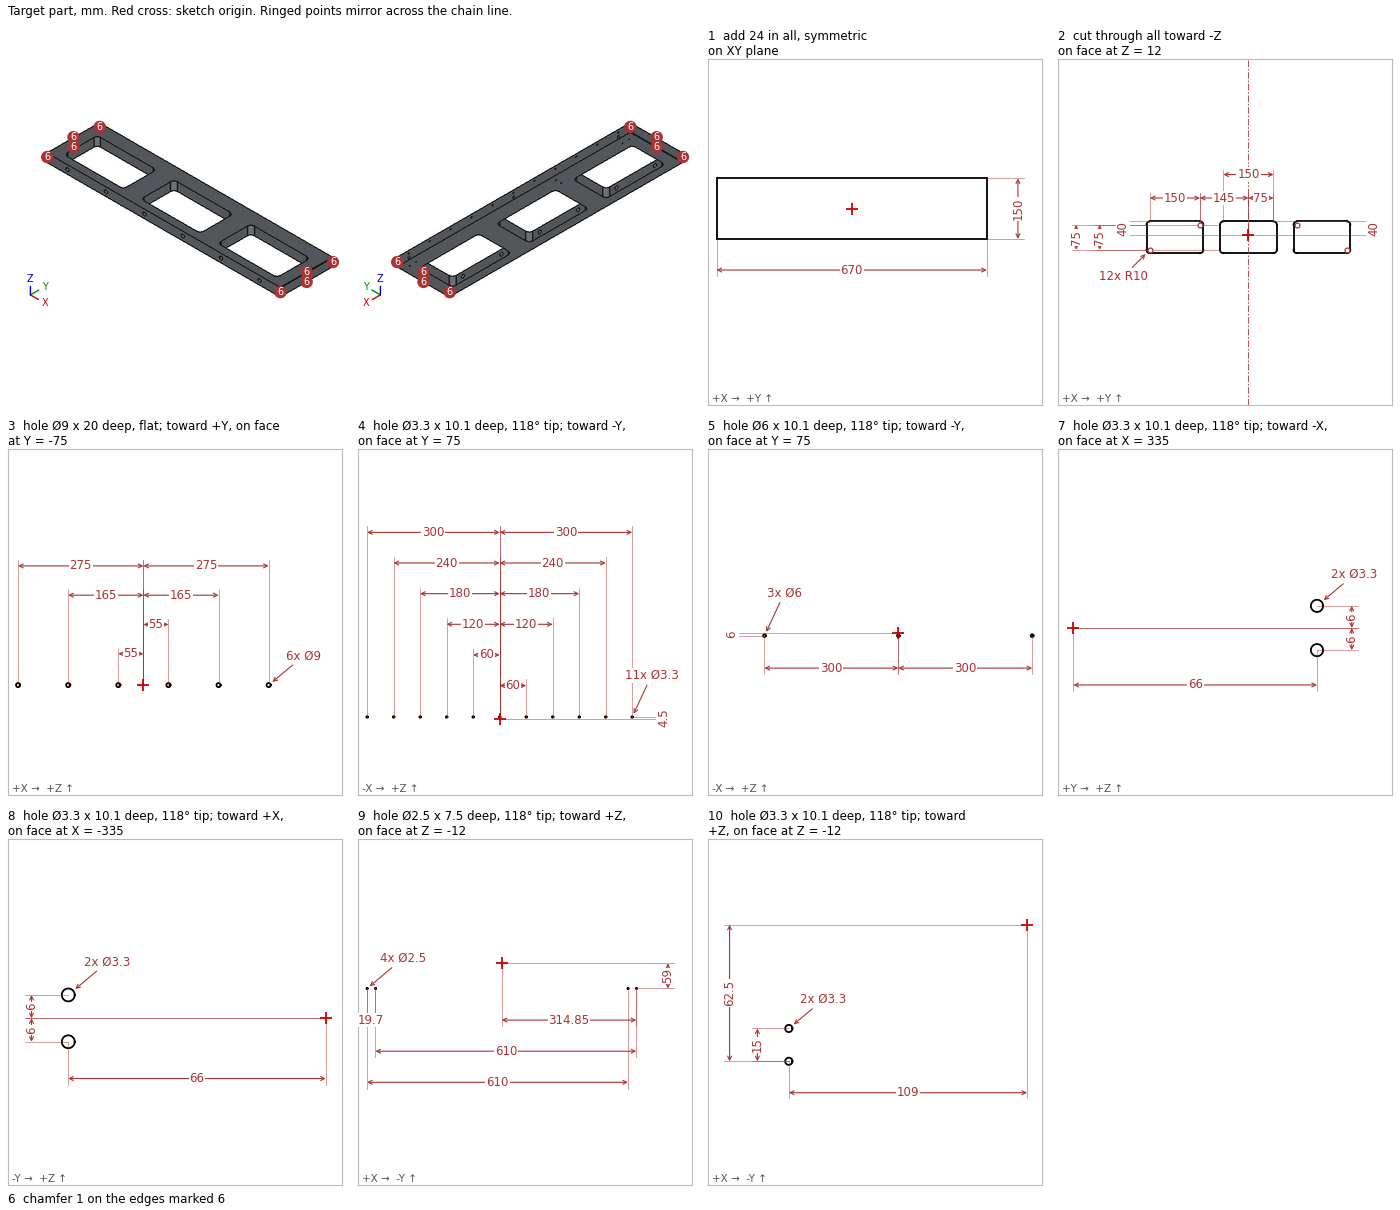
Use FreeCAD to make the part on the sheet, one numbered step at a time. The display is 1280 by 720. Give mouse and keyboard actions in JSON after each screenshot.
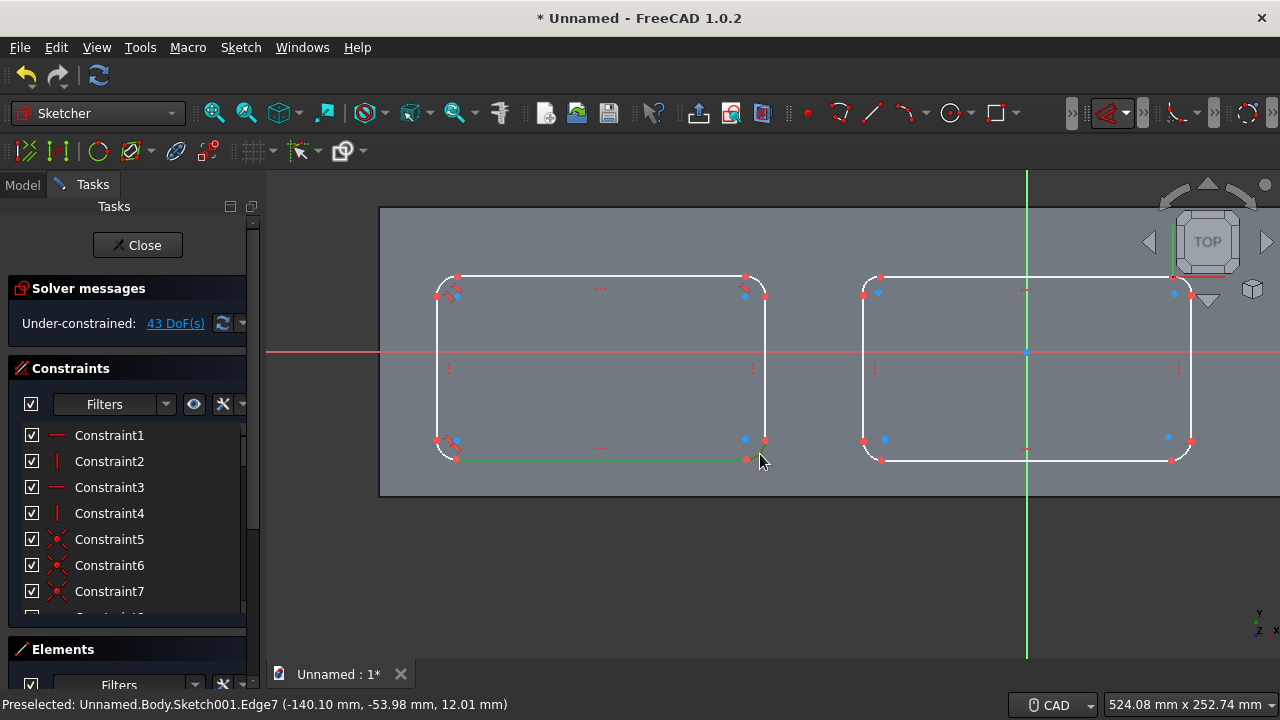
{"action": "key", "text": "t"}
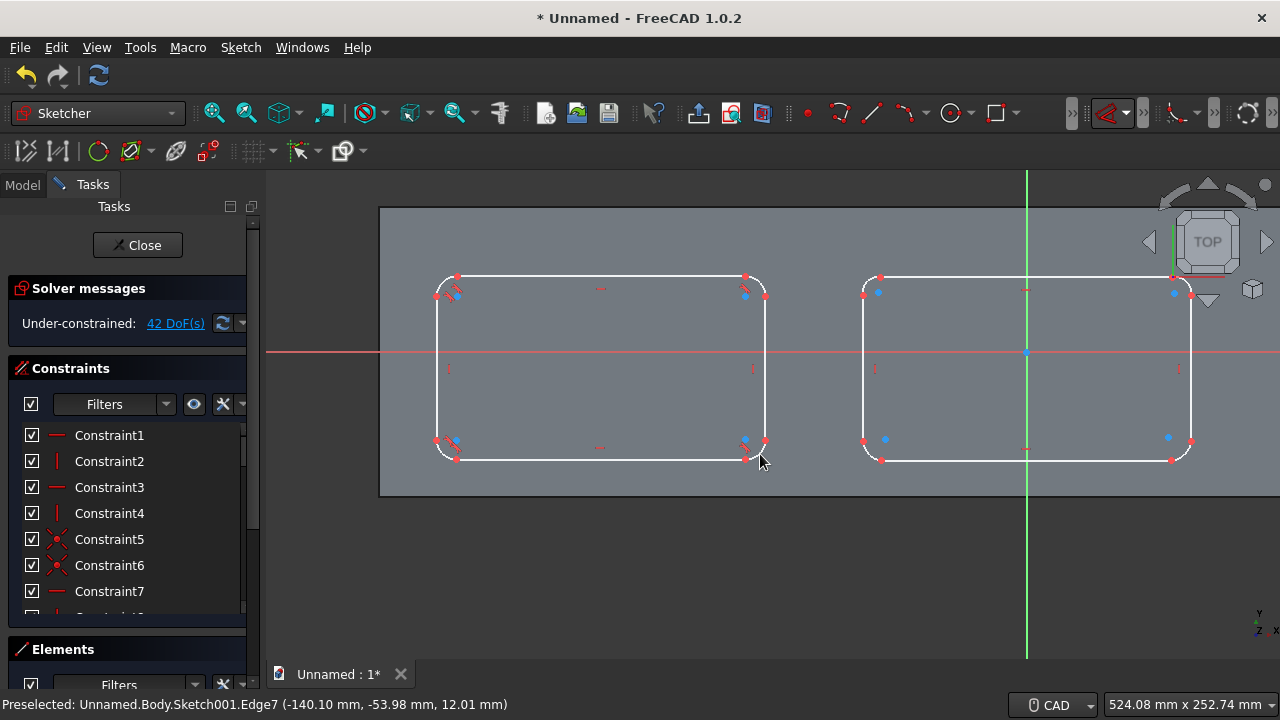
{"action": "left_click", "coordinate": [765, 397]}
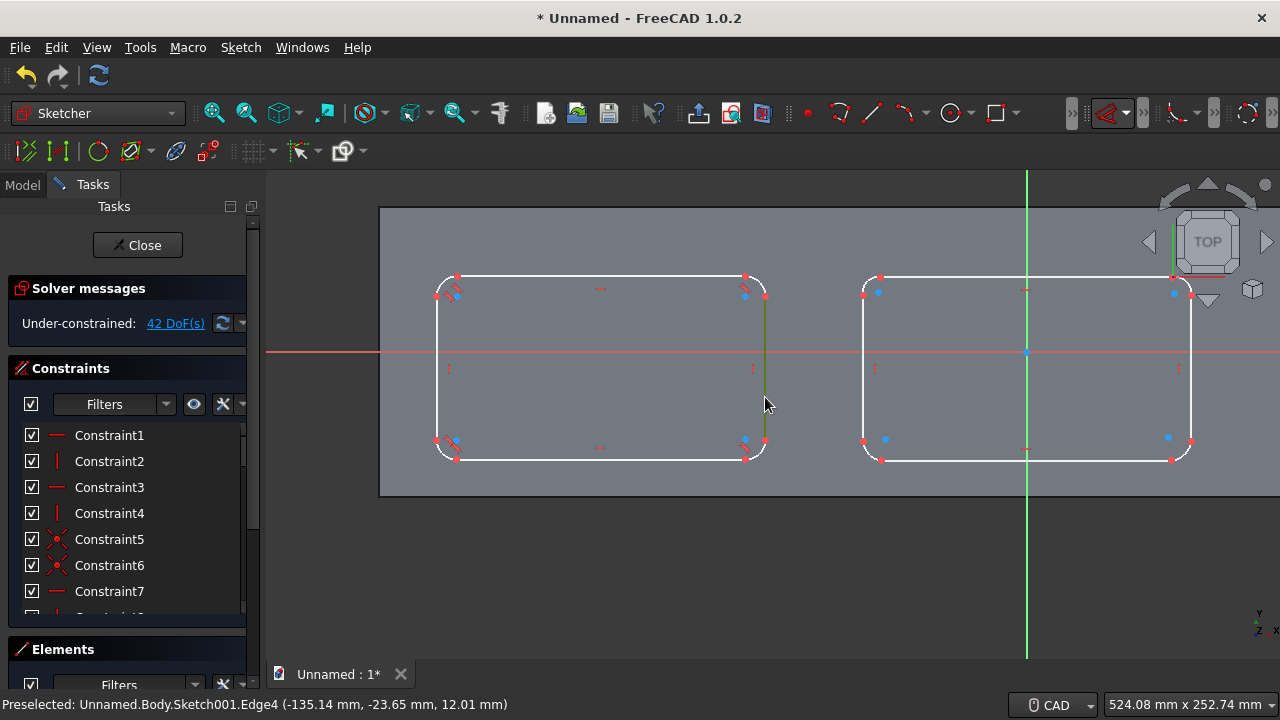
{"action": "scroll", "coordinate": [754, 457], "scroll_direction": "up", "scroll_amount": 3}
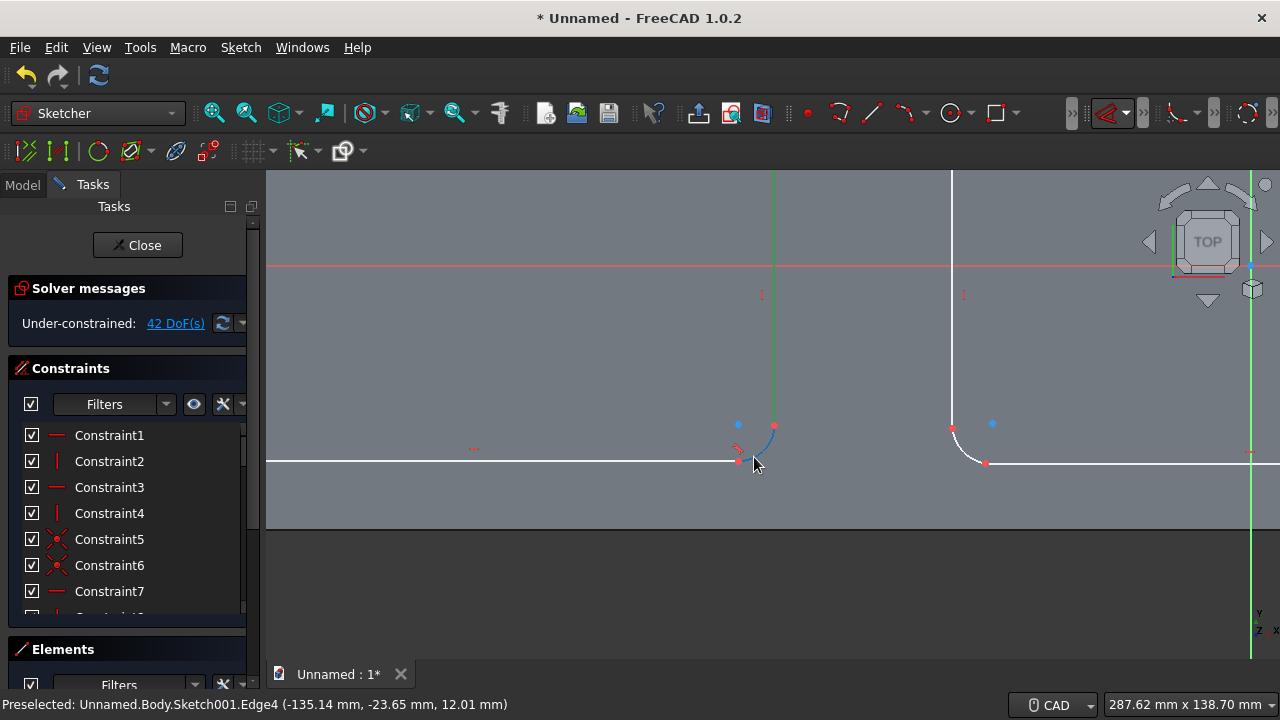
{"action": "left_click", "coordinate": [754, 457]}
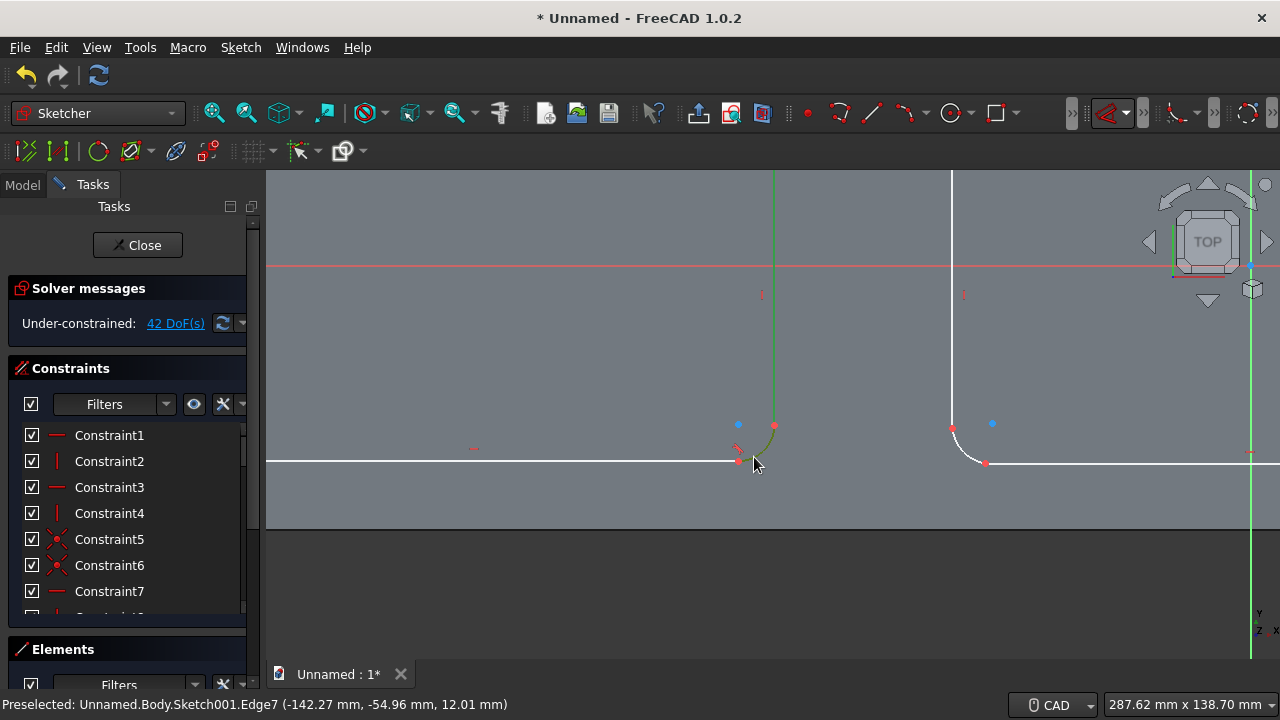
{"action": "key", "text": "t"}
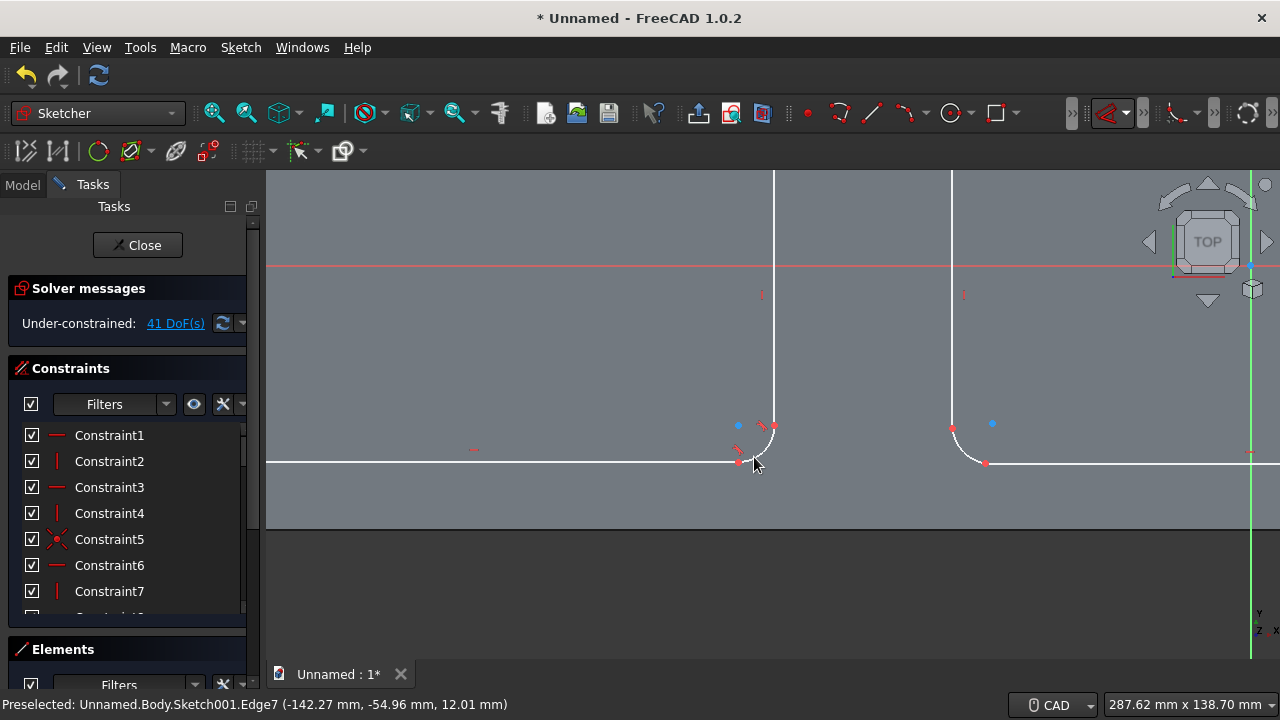
{"action": "scroll", "coordinate": [526, 455], "scroll_direction": "down", "scroll_amount": 7}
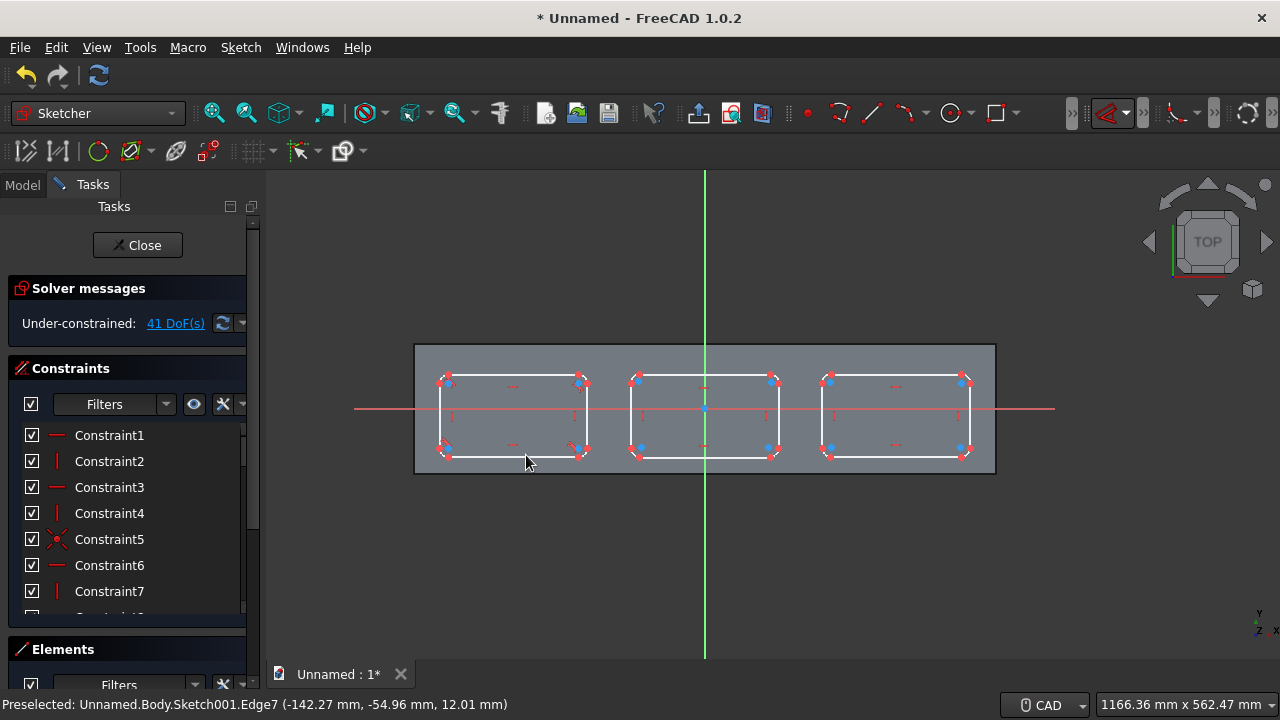
{"action": "left_click", "coordinate": [587, 429]}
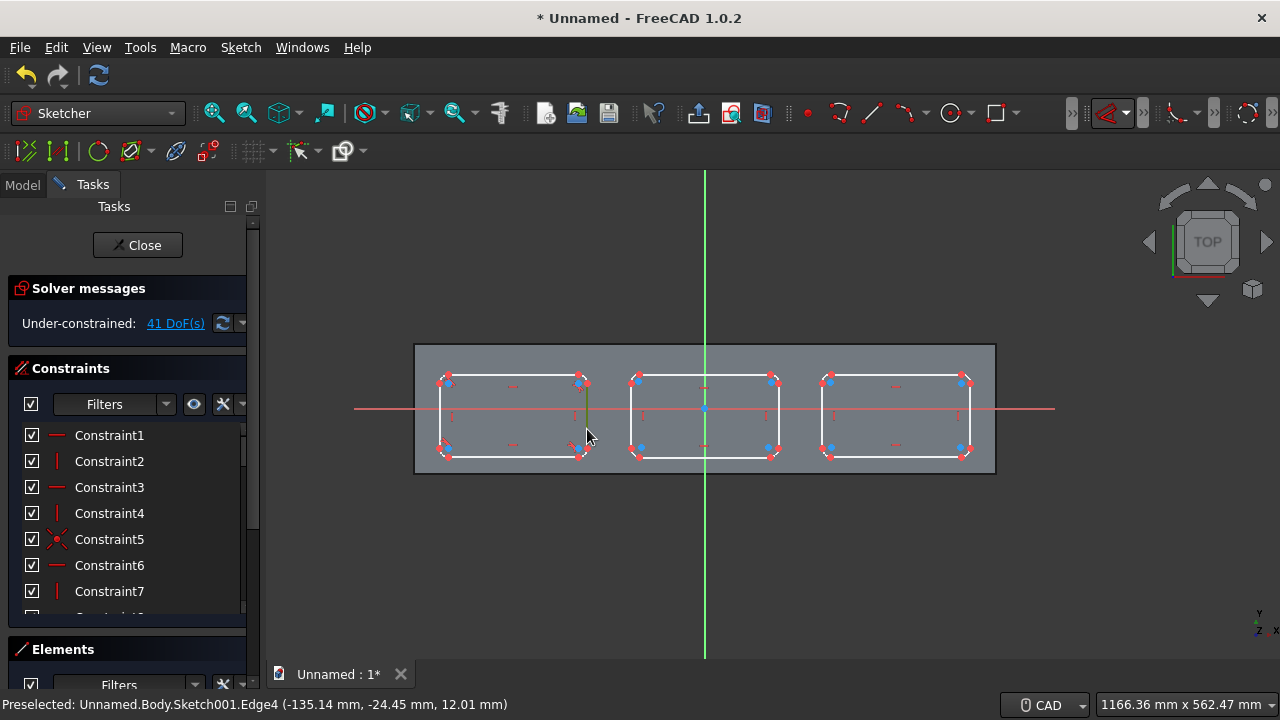
{"action": "scroll", "coordinate": [585, 377], "scroll_direction": "up", "scroll_amount": 4}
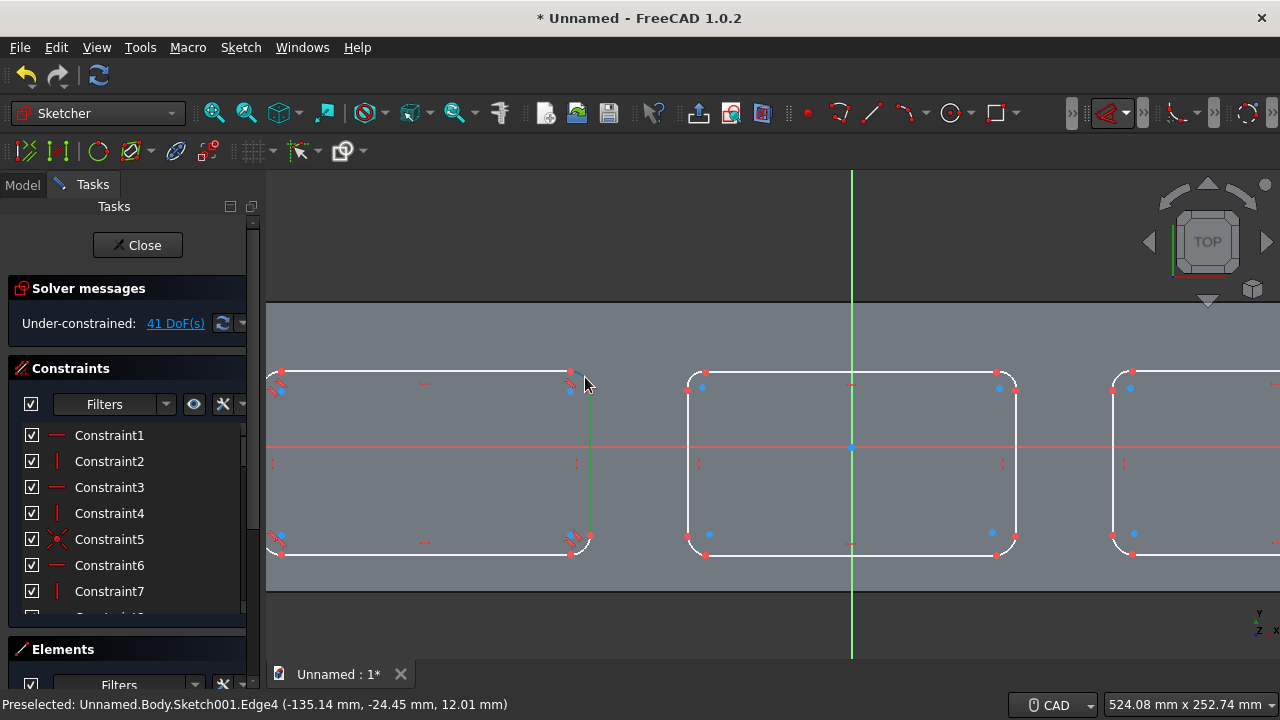
{"action": "left_click", "coordinate": [584, 377]}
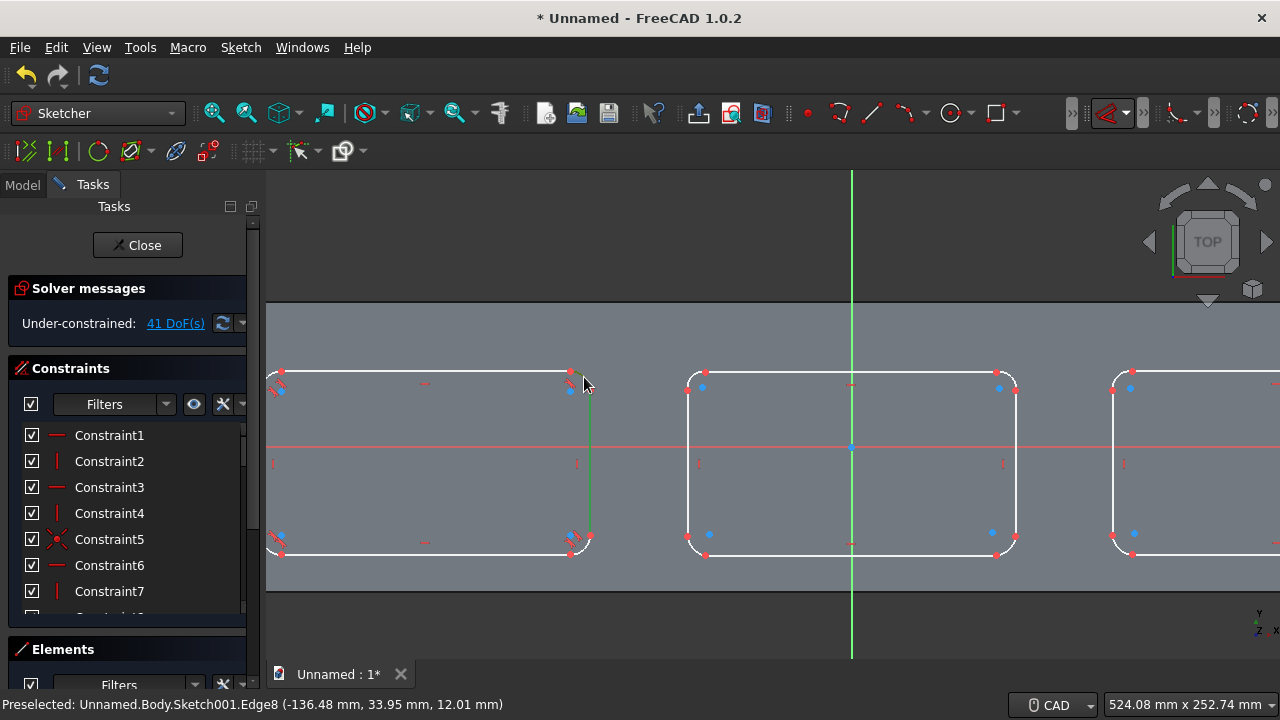
{"action": "key", "text": "t"}